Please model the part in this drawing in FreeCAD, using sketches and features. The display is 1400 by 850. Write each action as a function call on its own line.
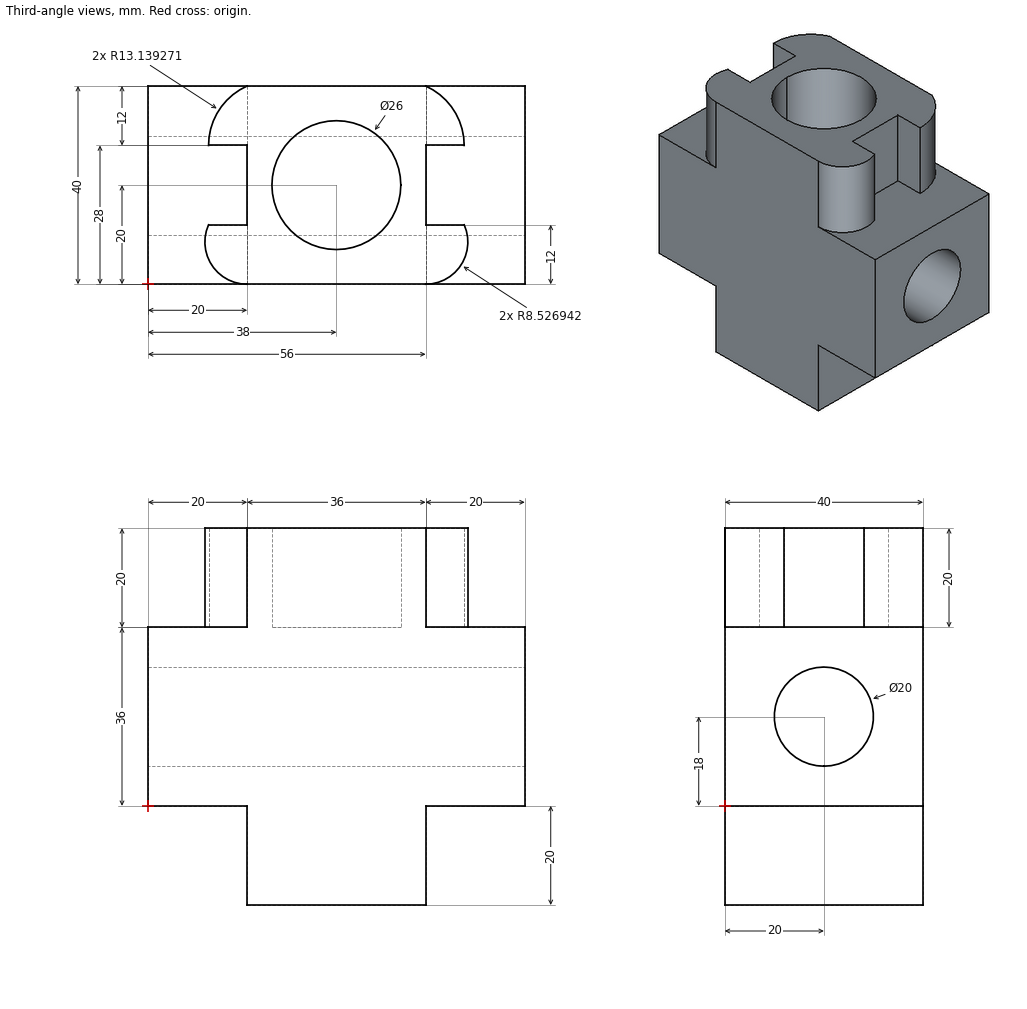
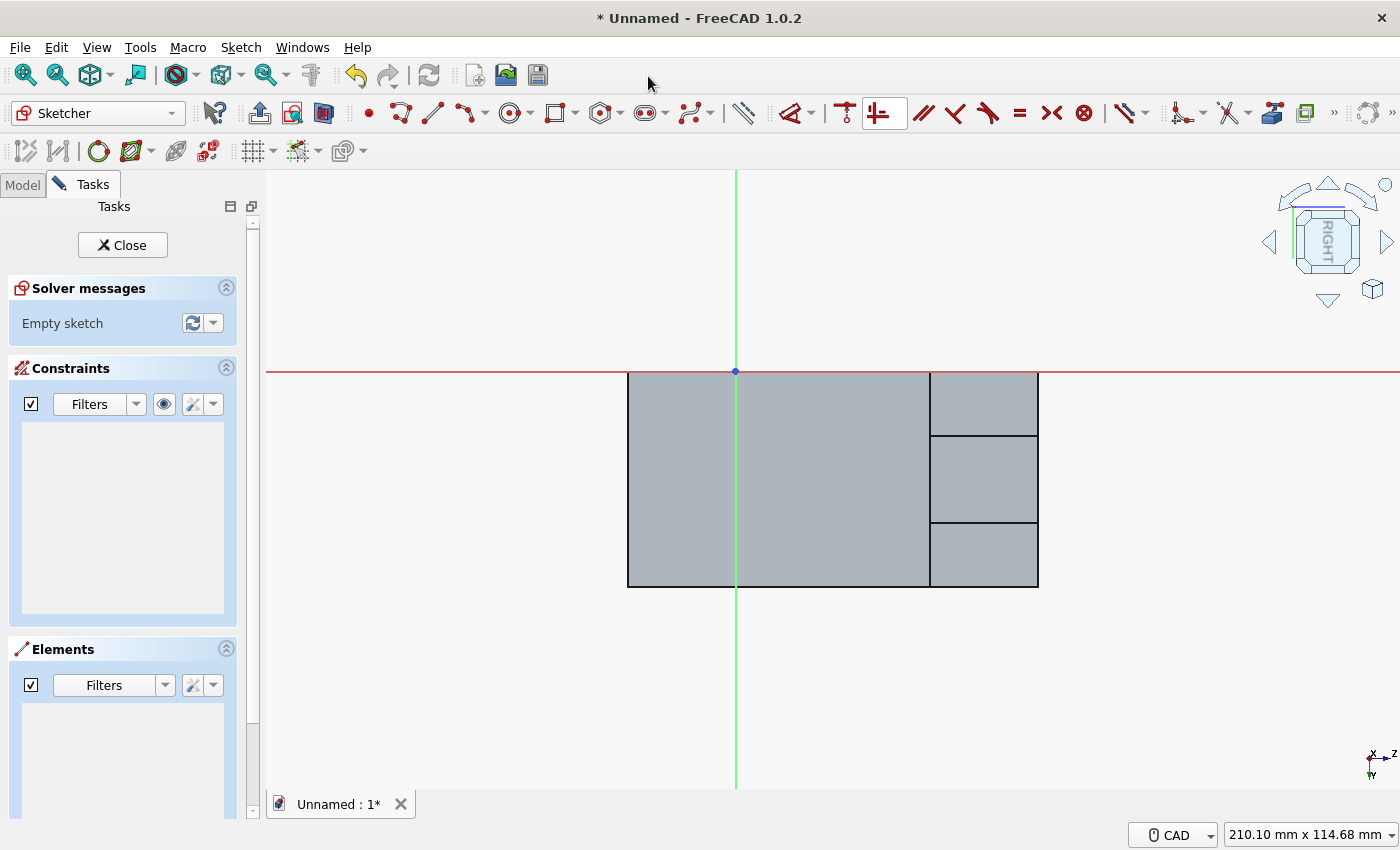
scroll(850, 430, up, 4)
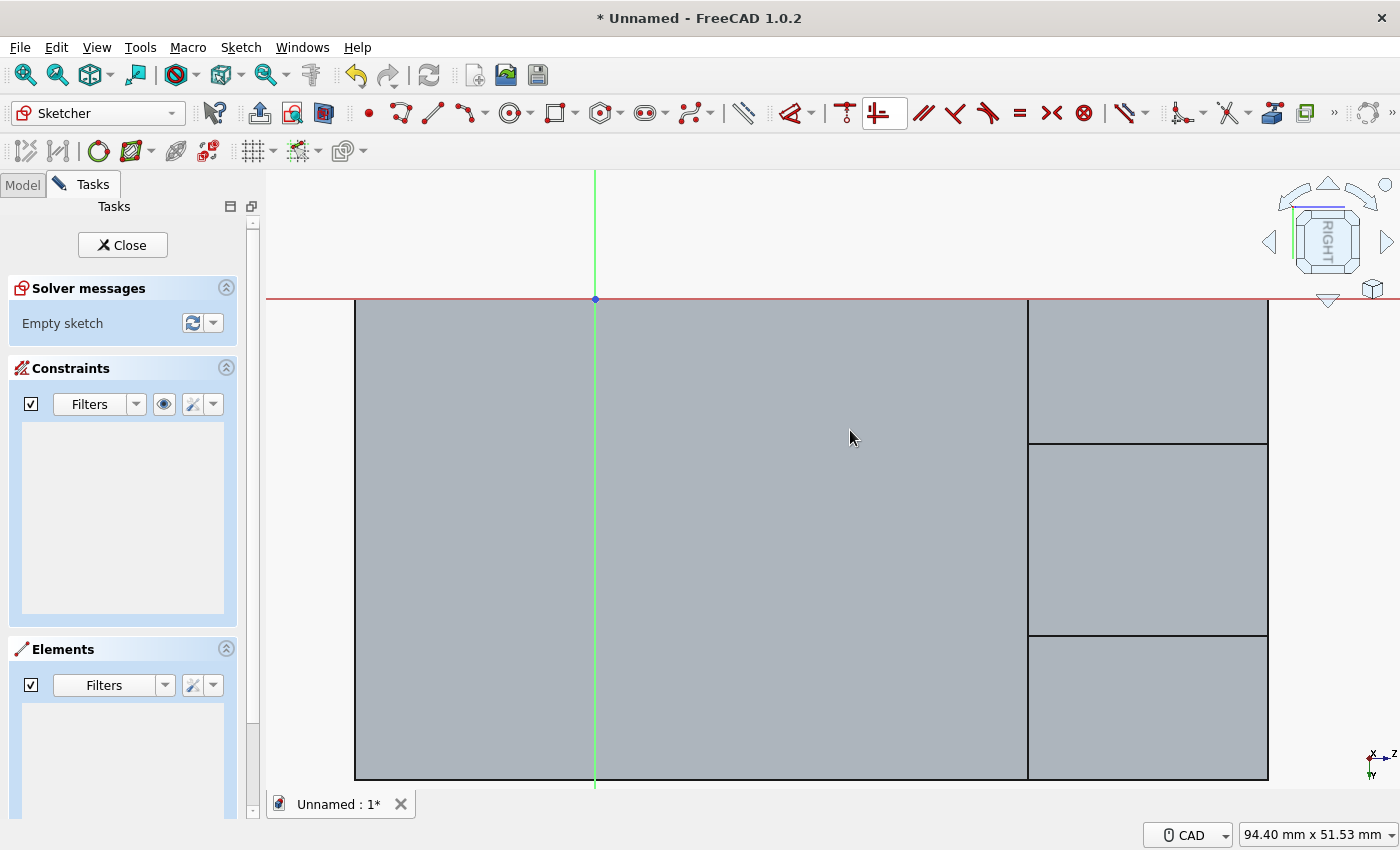
click(510, 114)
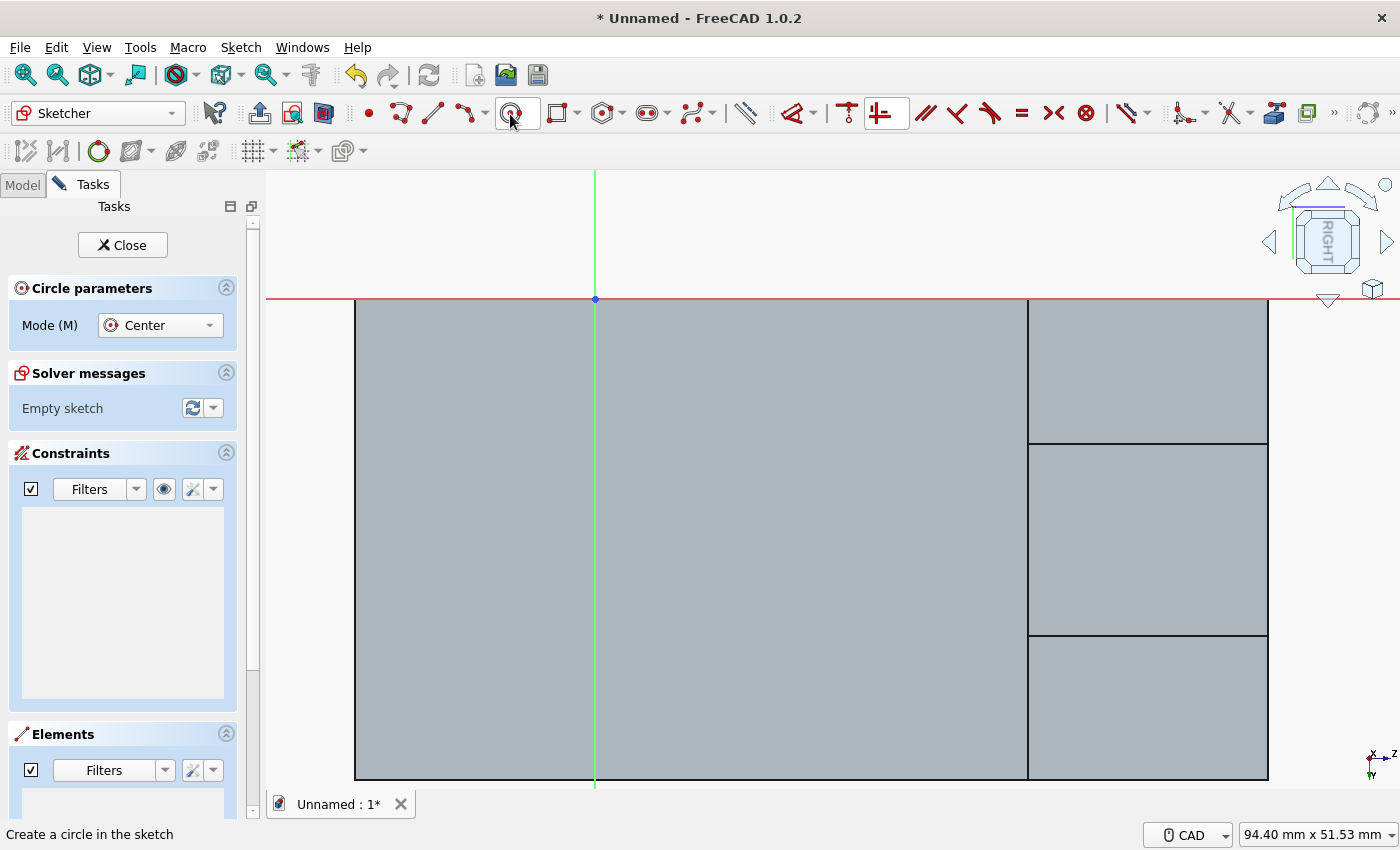
click(812, 540)
move(896, 455)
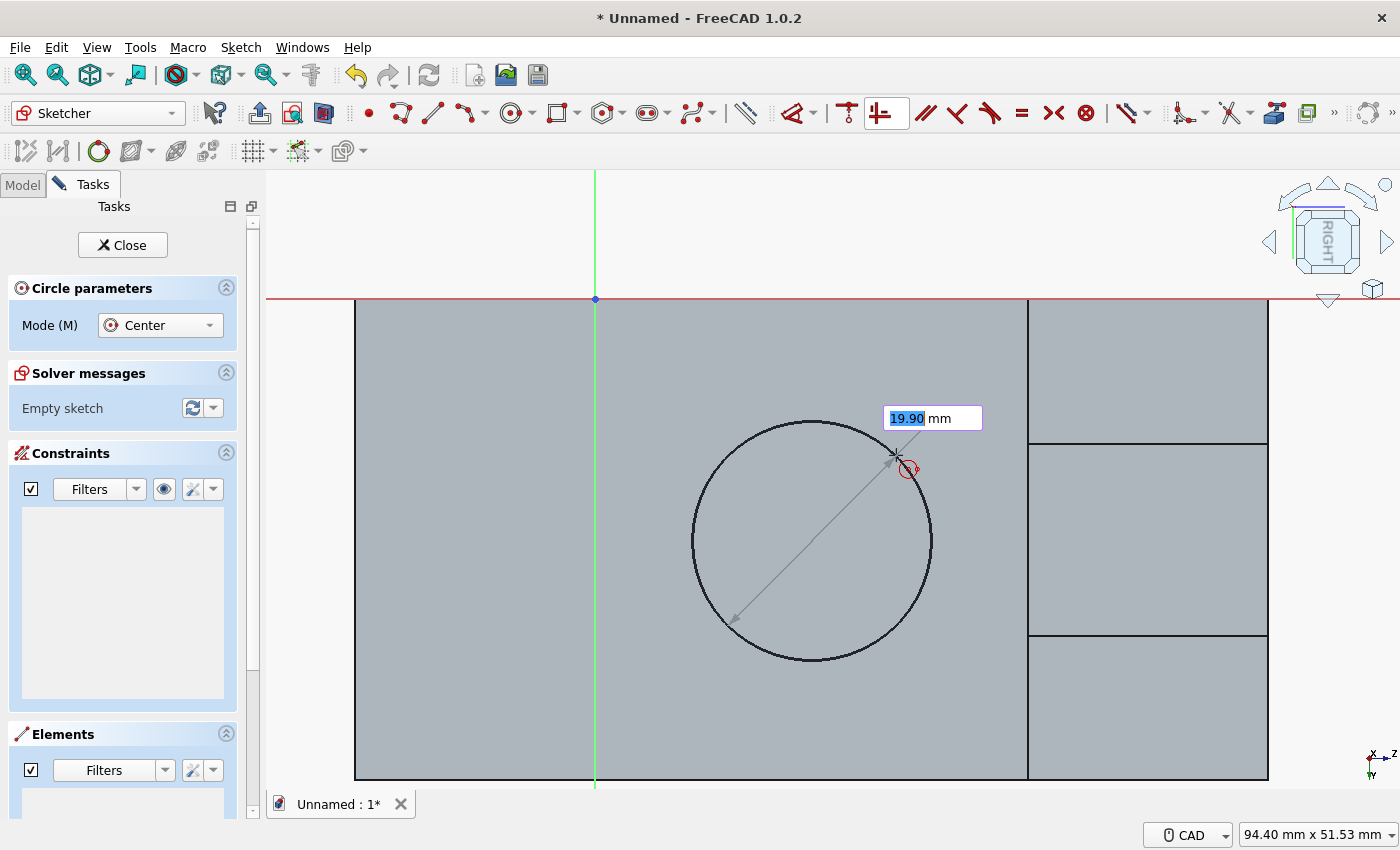
text(20)
key(Return)
key(Escape)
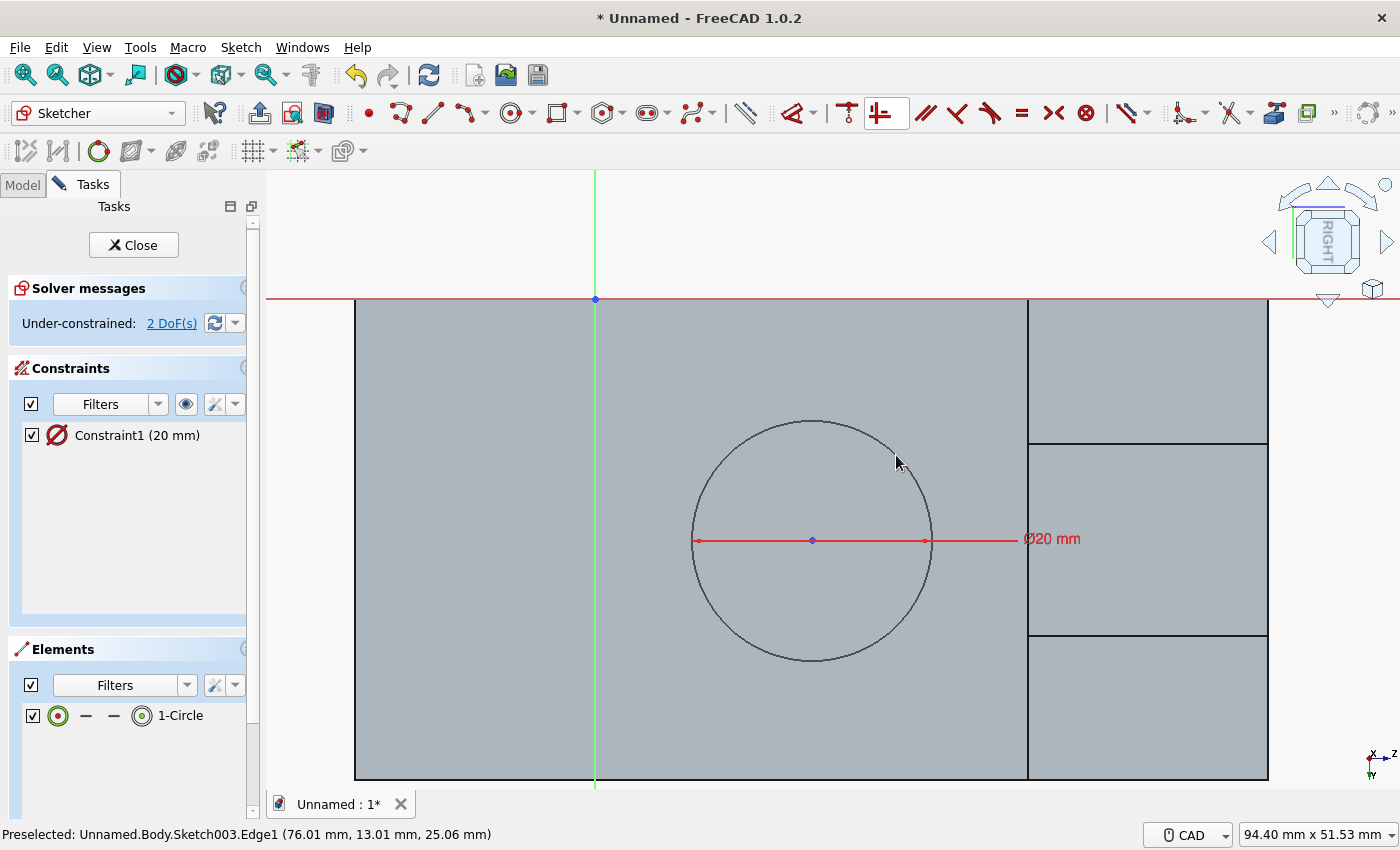
click(792, 114)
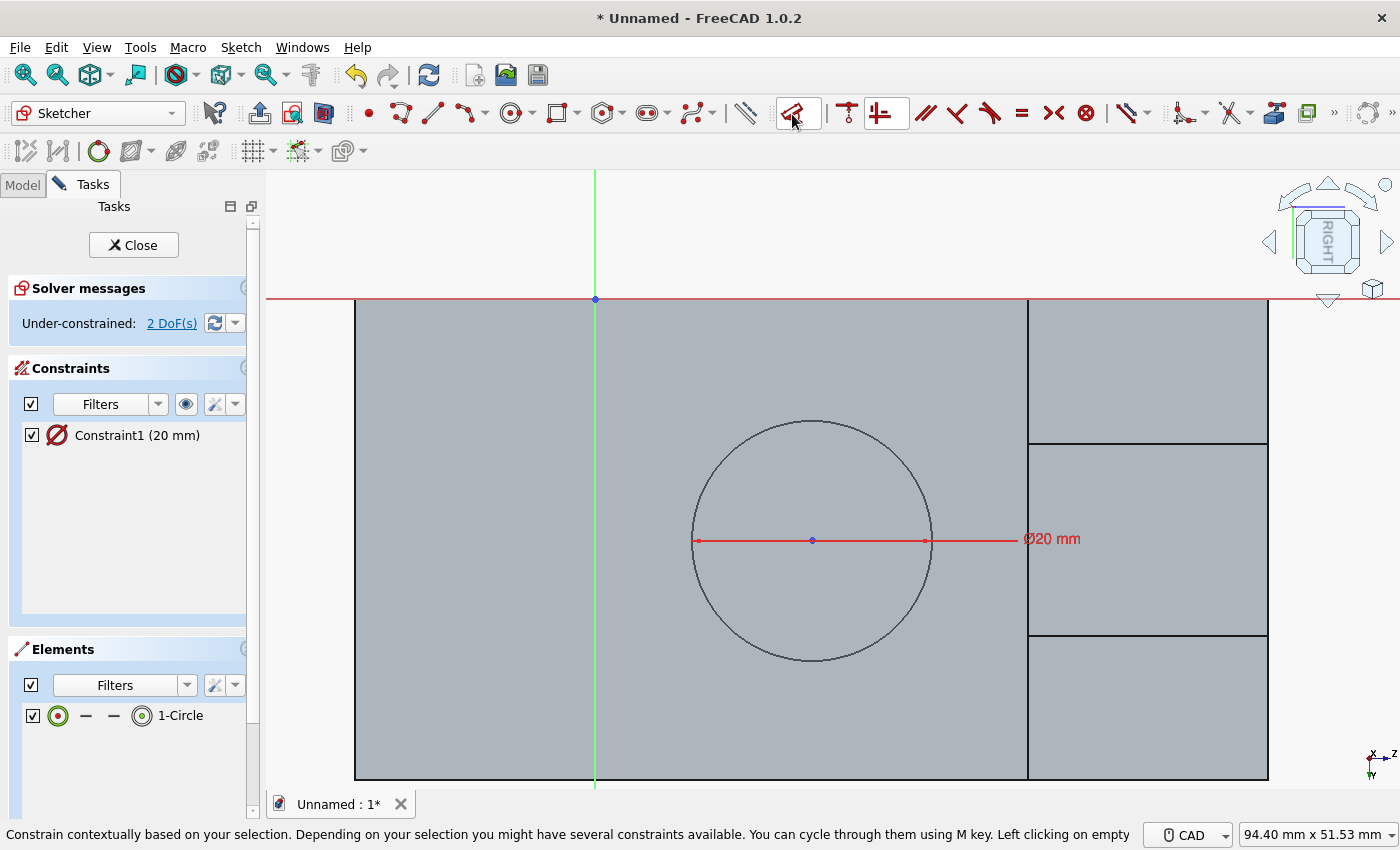
click(812, 541)
click(704, 265)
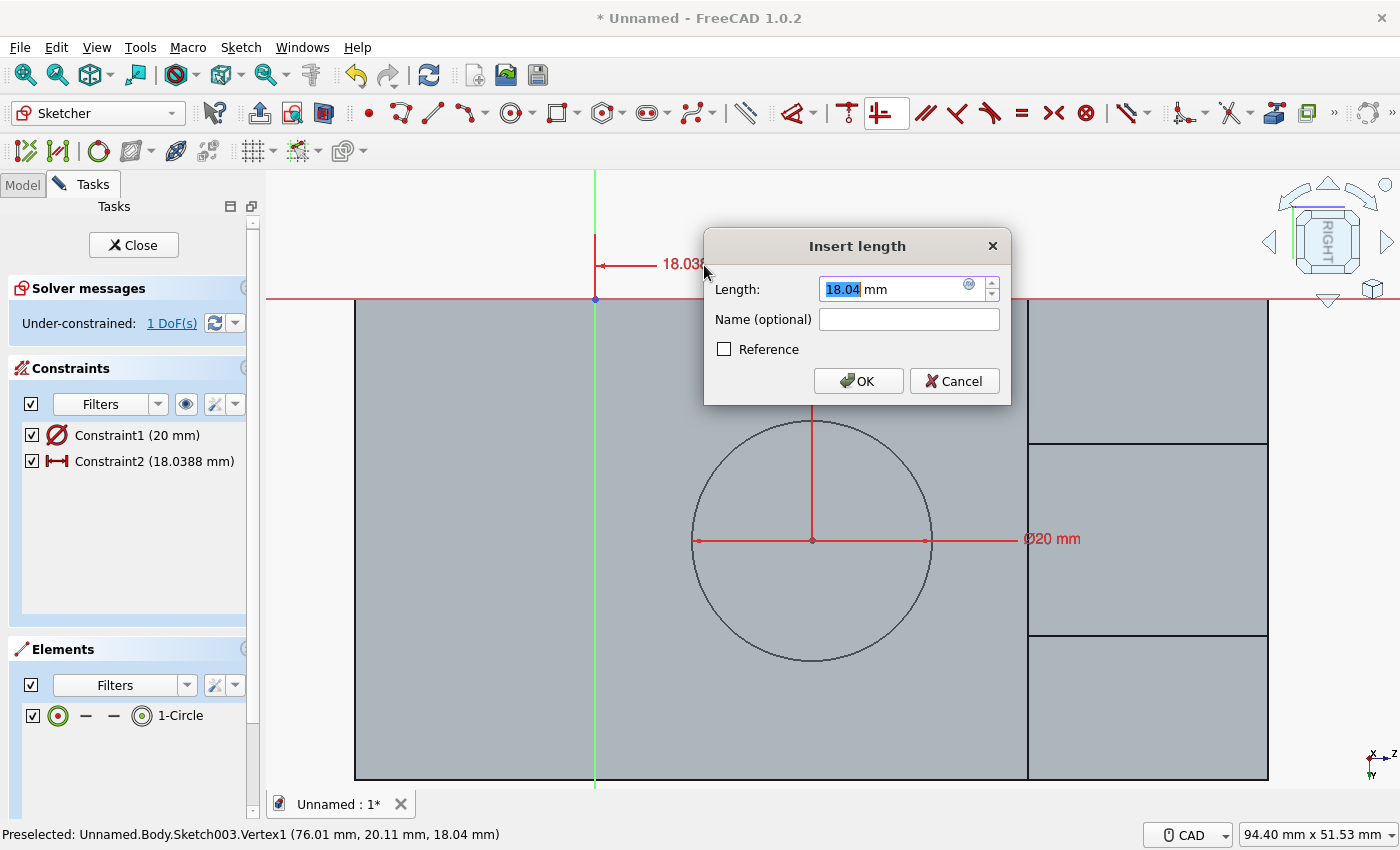
text(18)
key(Return)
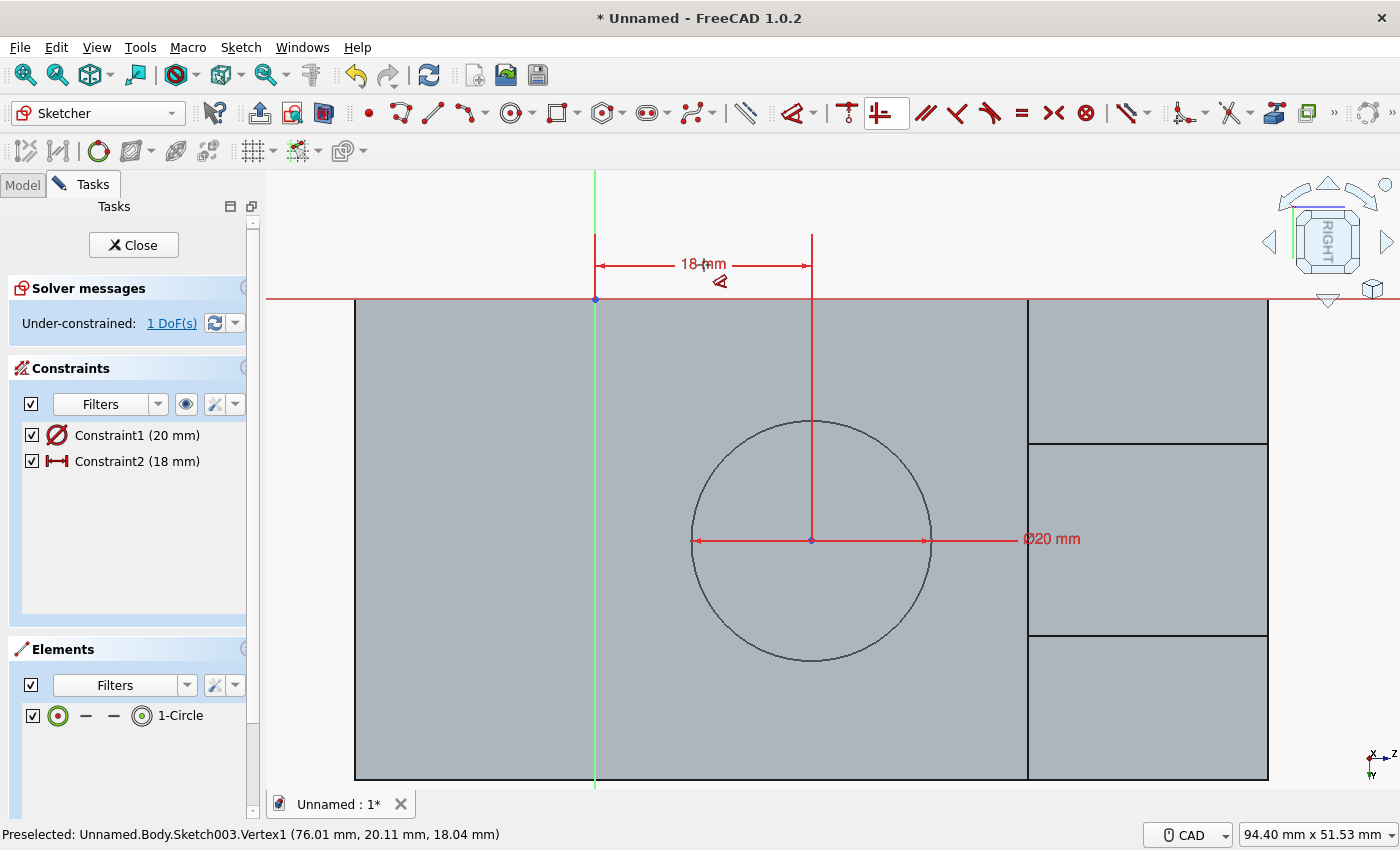
click(812, 541)
click(561, 420)